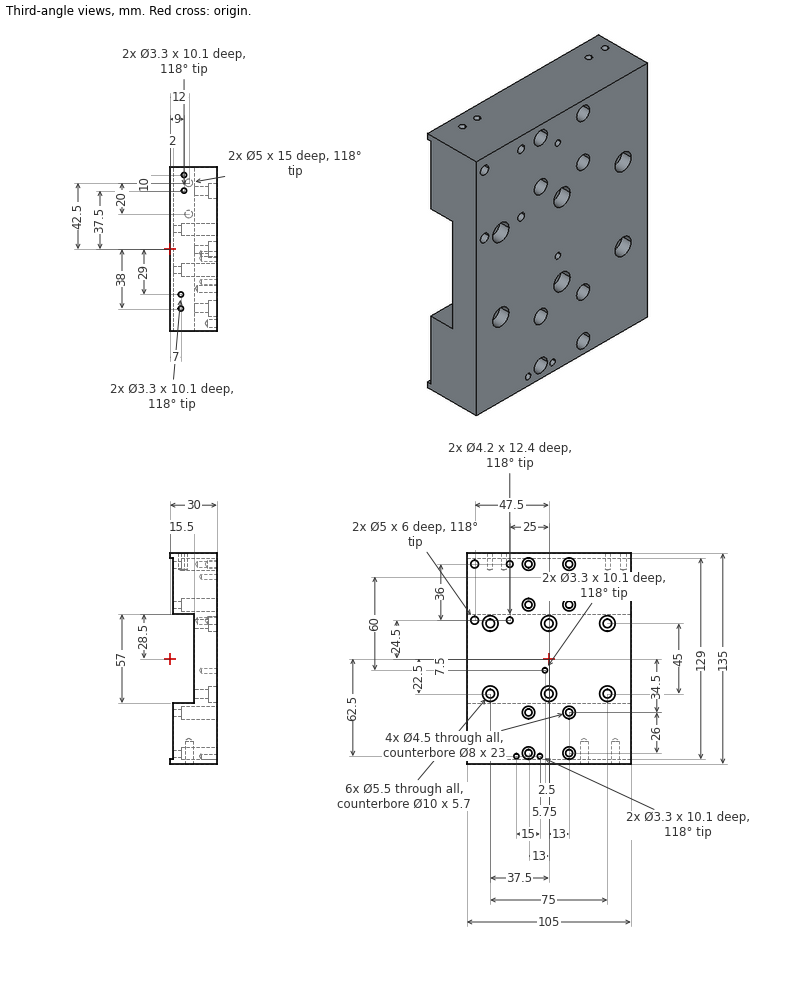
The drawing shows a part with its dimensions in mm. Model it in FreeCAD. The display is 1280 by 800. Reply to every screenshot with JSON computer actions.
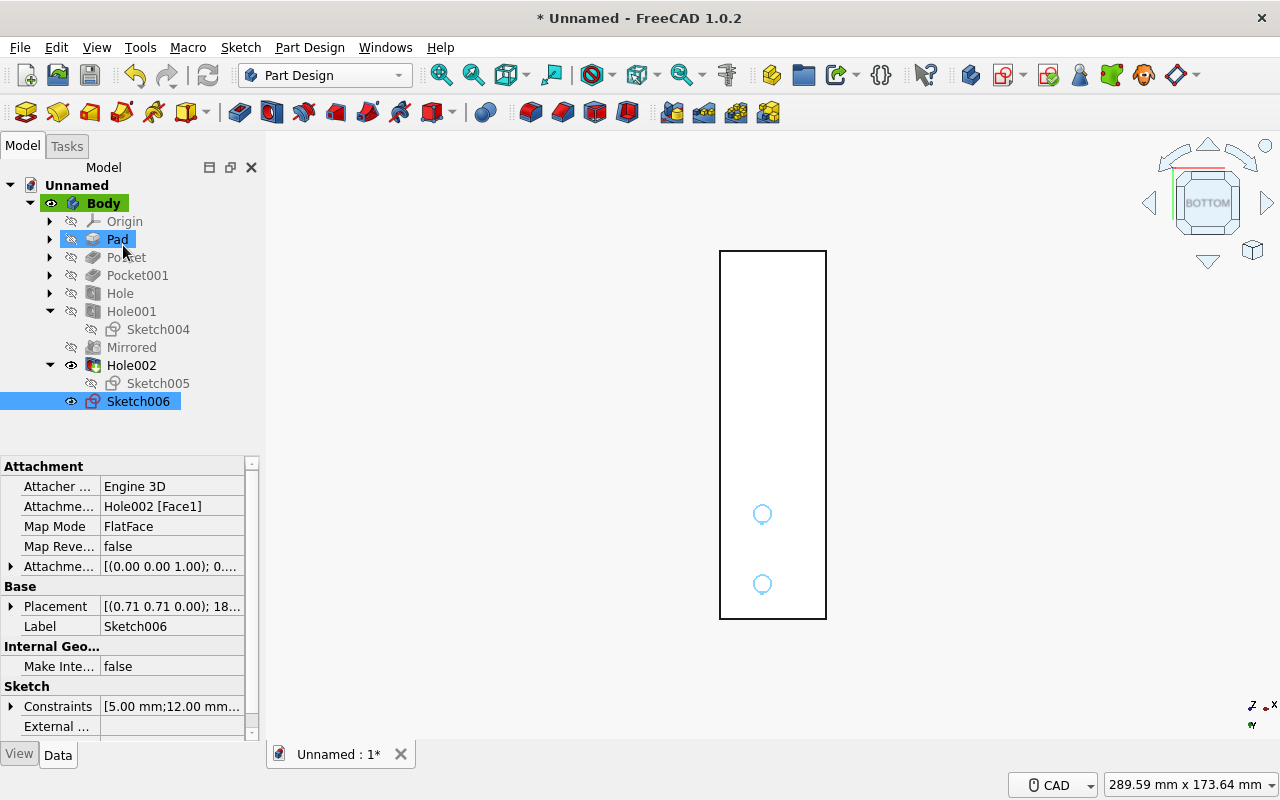
{"action": "left_click", "coordinate": [272, 112]}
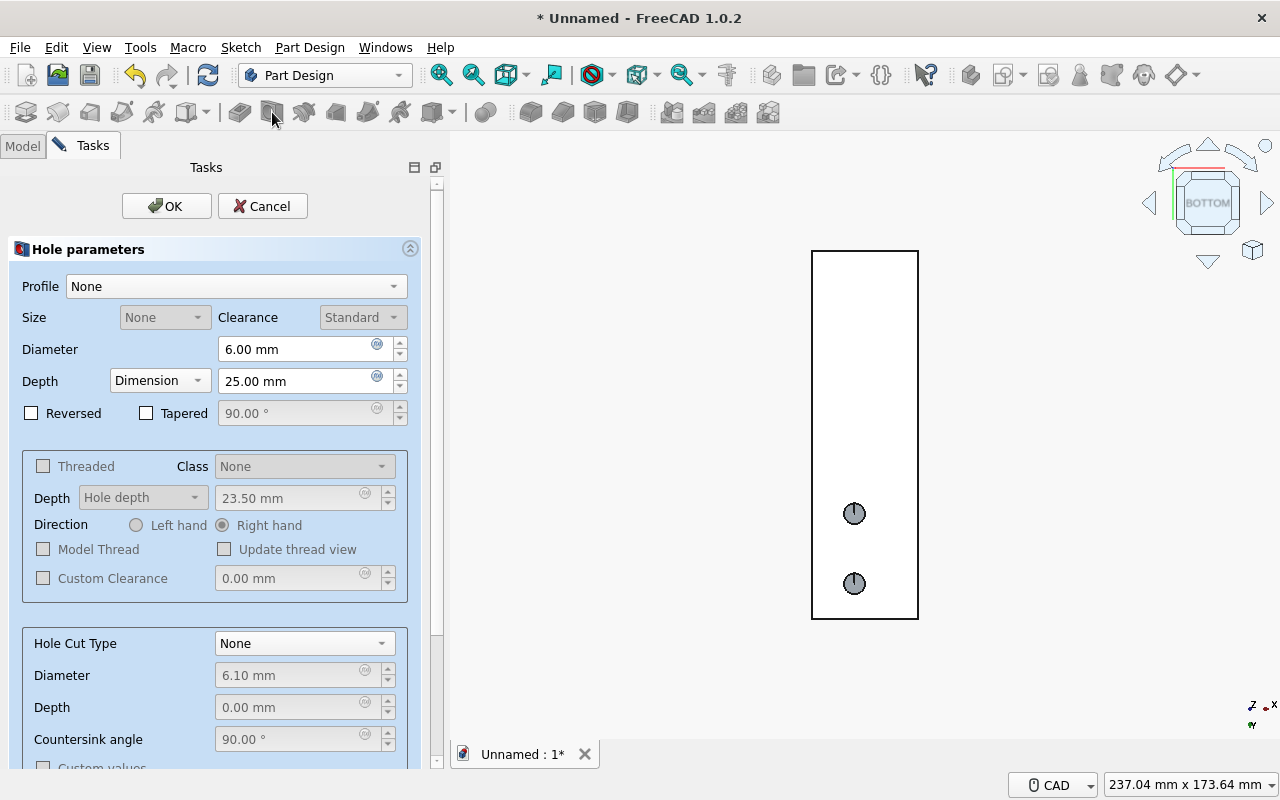
{"action": "triple_click", "coordinate": [305, 349]}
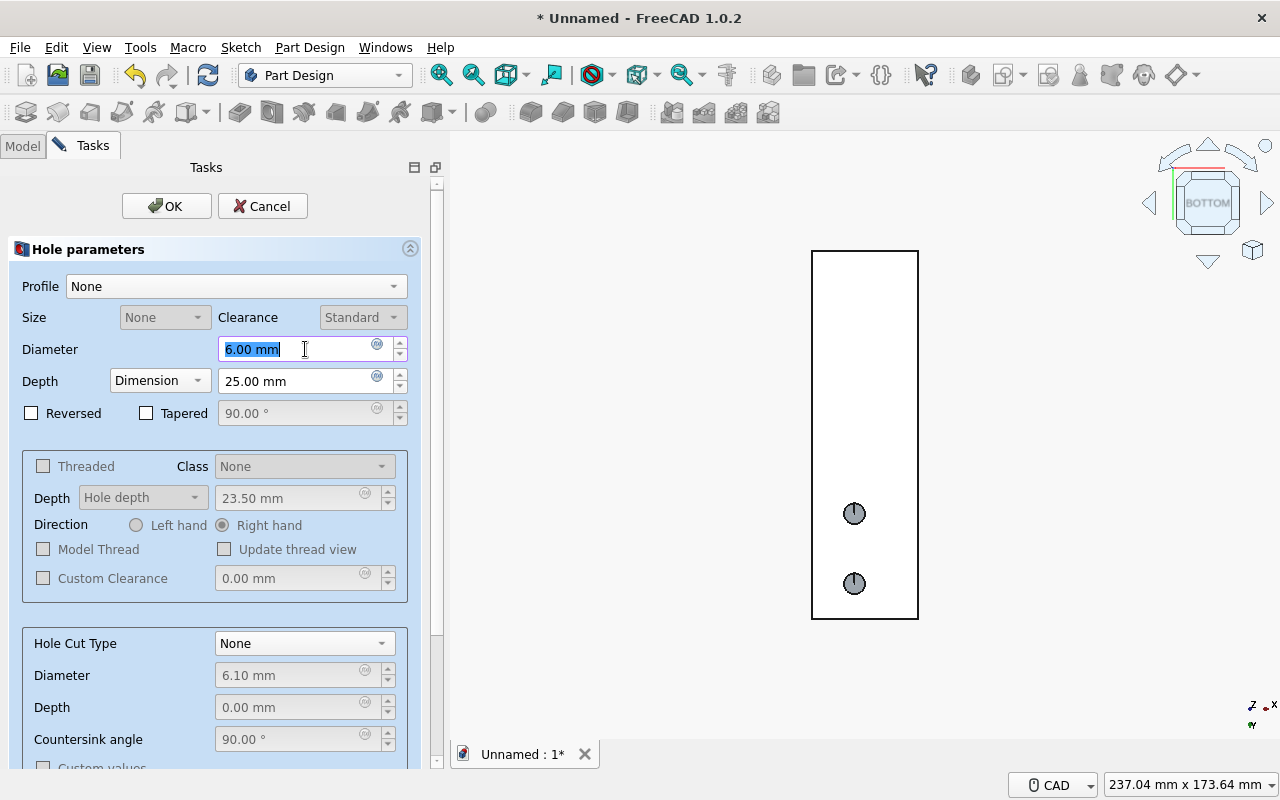
{"action": "type", "text": "5"}
{"action": "key", "text": "Tab"}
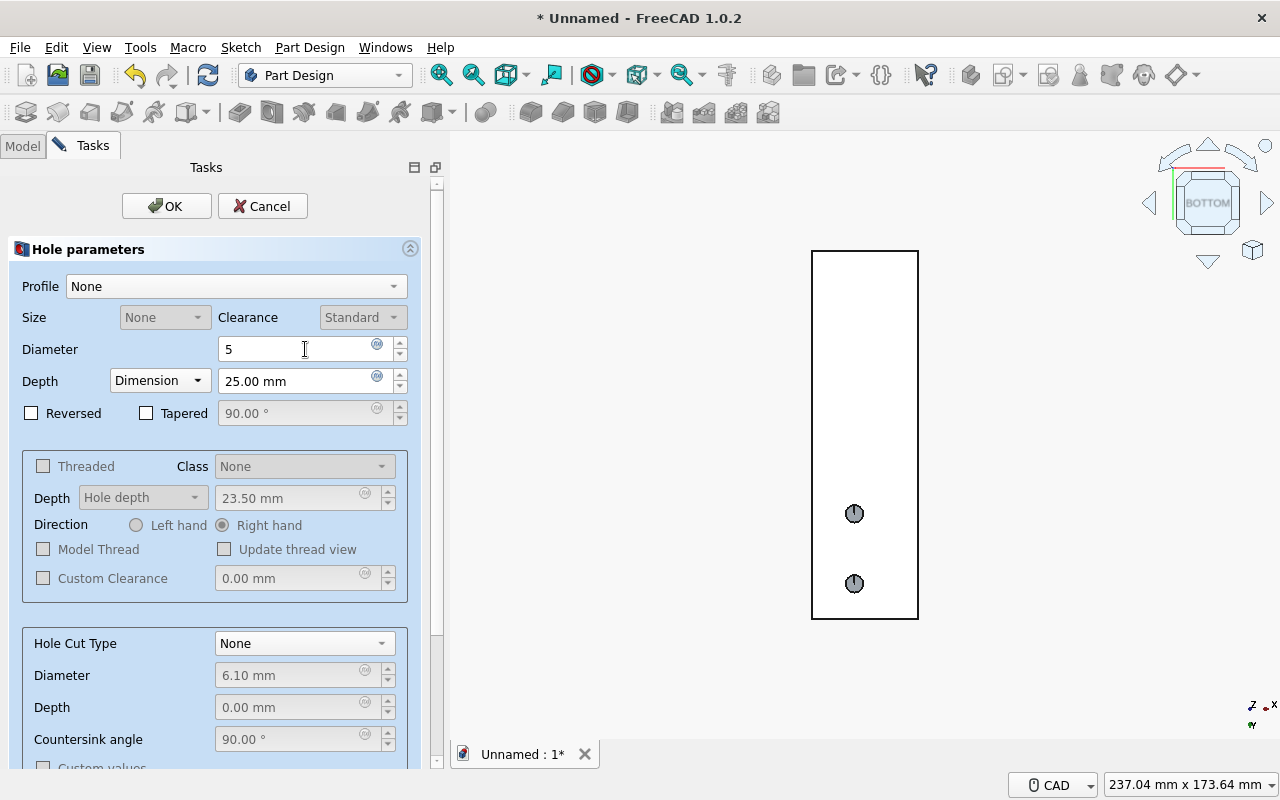
{"action": "triple_click", "coordinate": [305, 381]}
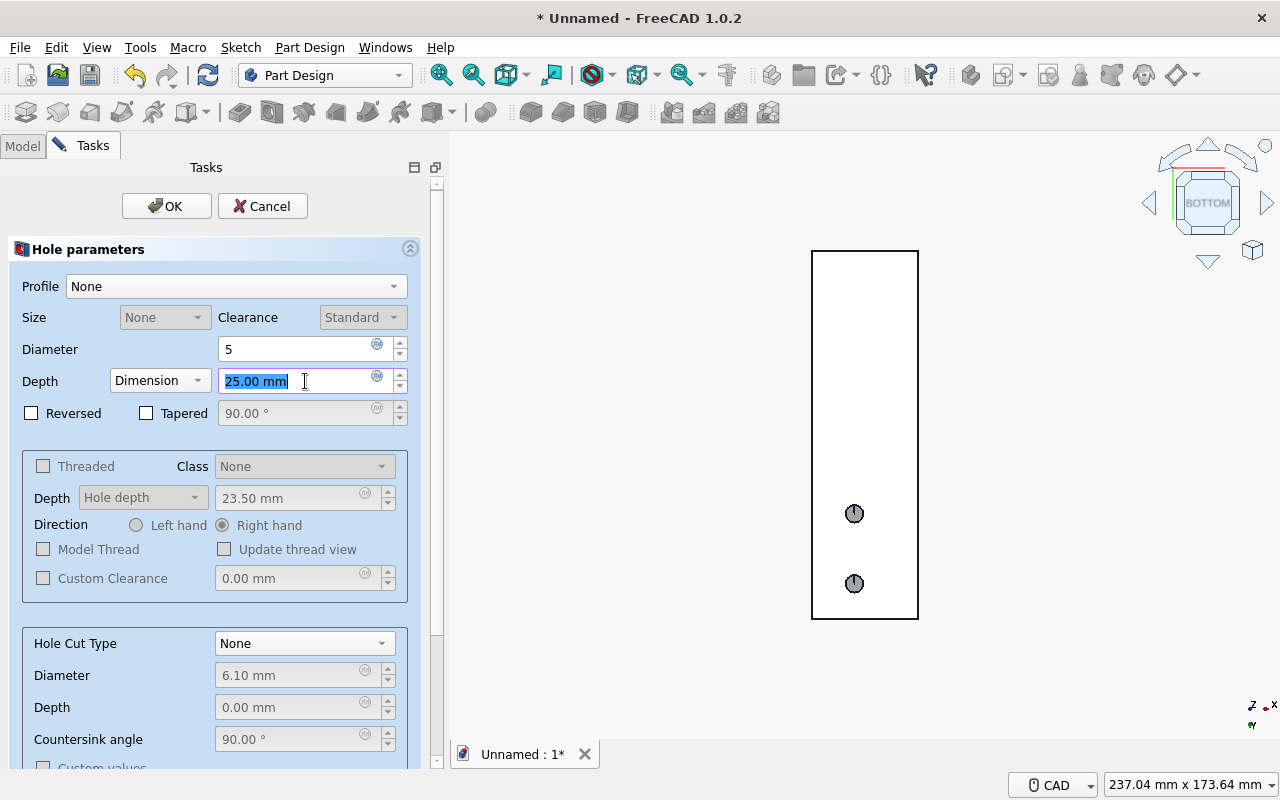
{"action": "type", "text": "15"}
{"action": "key", "text": "Tab"}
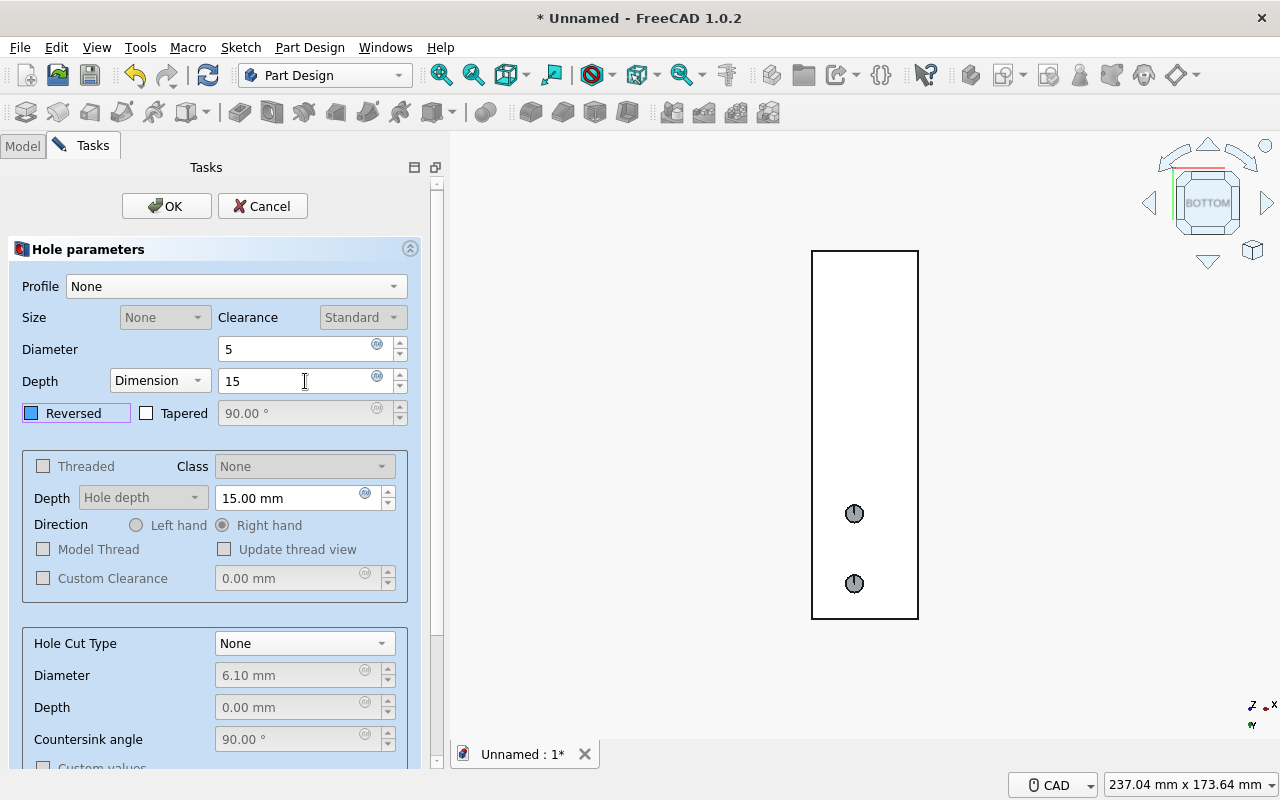
{"action": "left_click", "coordinate": [167, 206]}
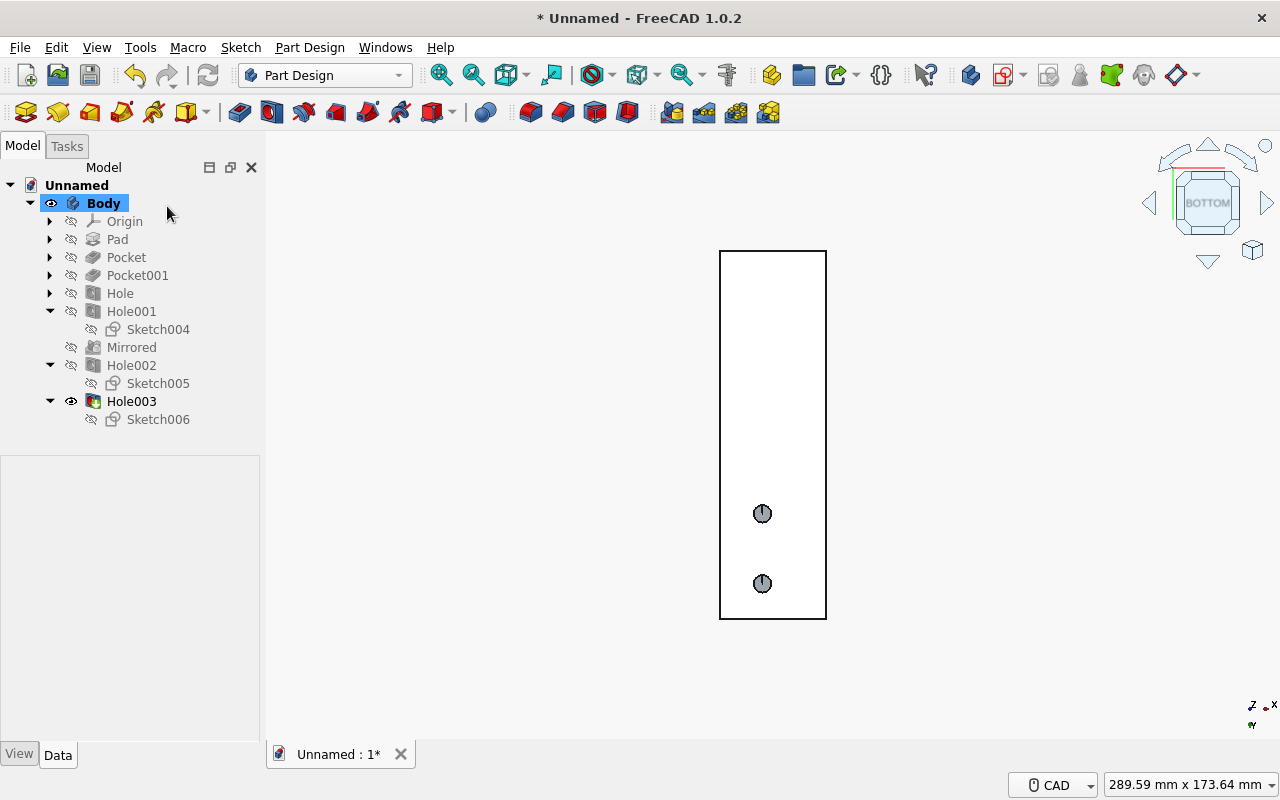
{"action": "key", "text": "0"}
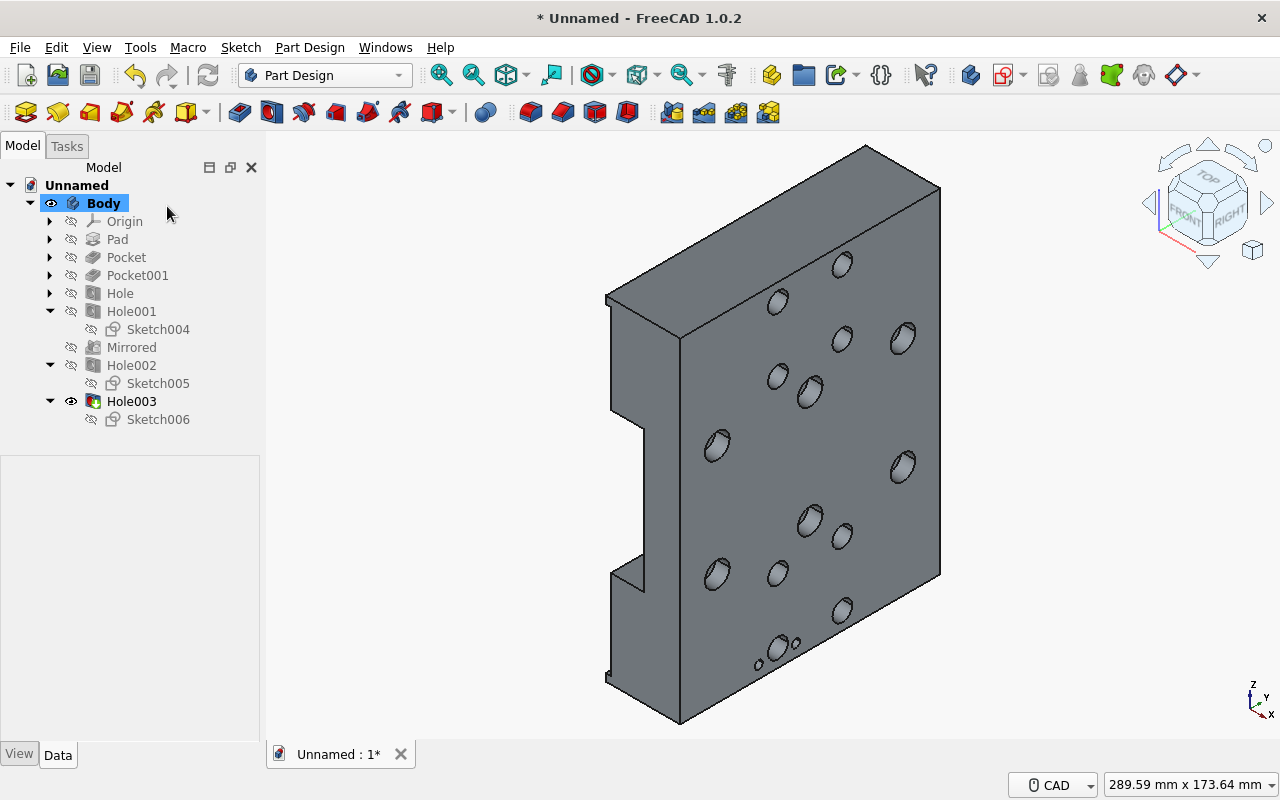
{"action": "left_click", "coordinate": [847, 198]}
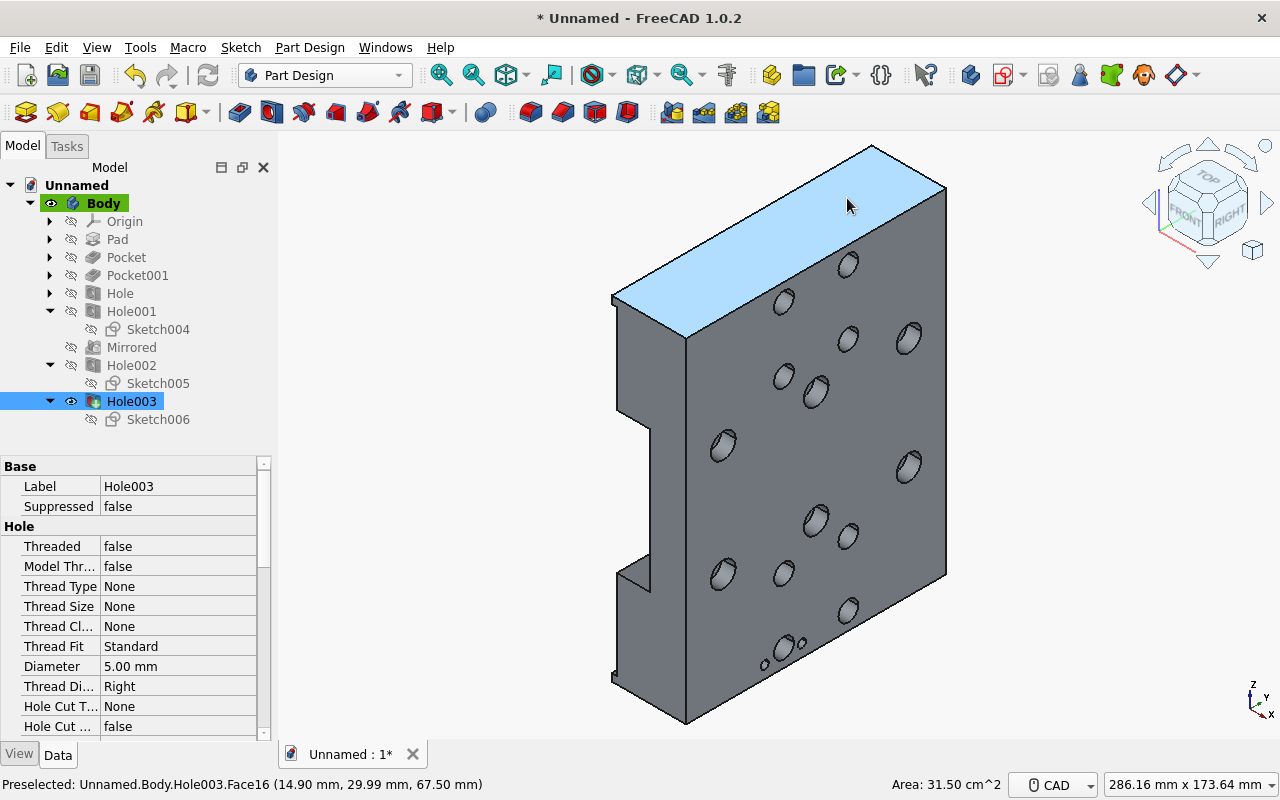
{"action": "left_click", "coordinate": [1004, 76]}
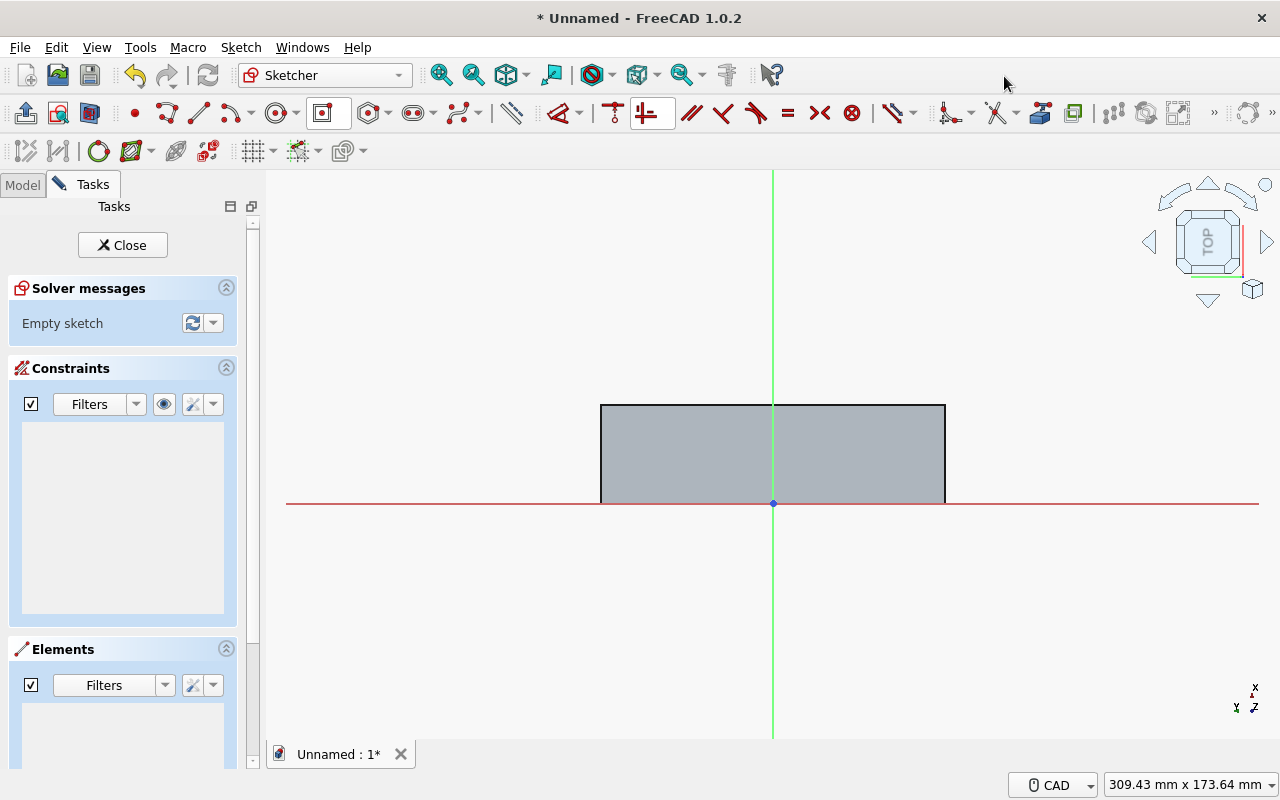
{"action": "scroll", "coordinate": [628, 476], "scroll_direction": "up", "scroll_amount": 13}